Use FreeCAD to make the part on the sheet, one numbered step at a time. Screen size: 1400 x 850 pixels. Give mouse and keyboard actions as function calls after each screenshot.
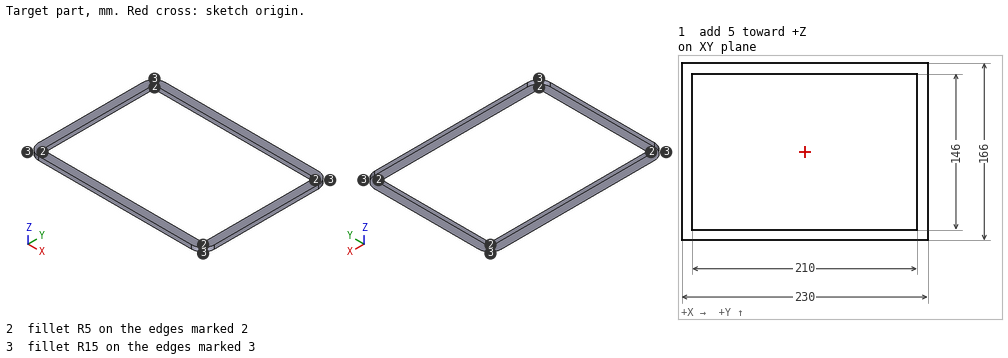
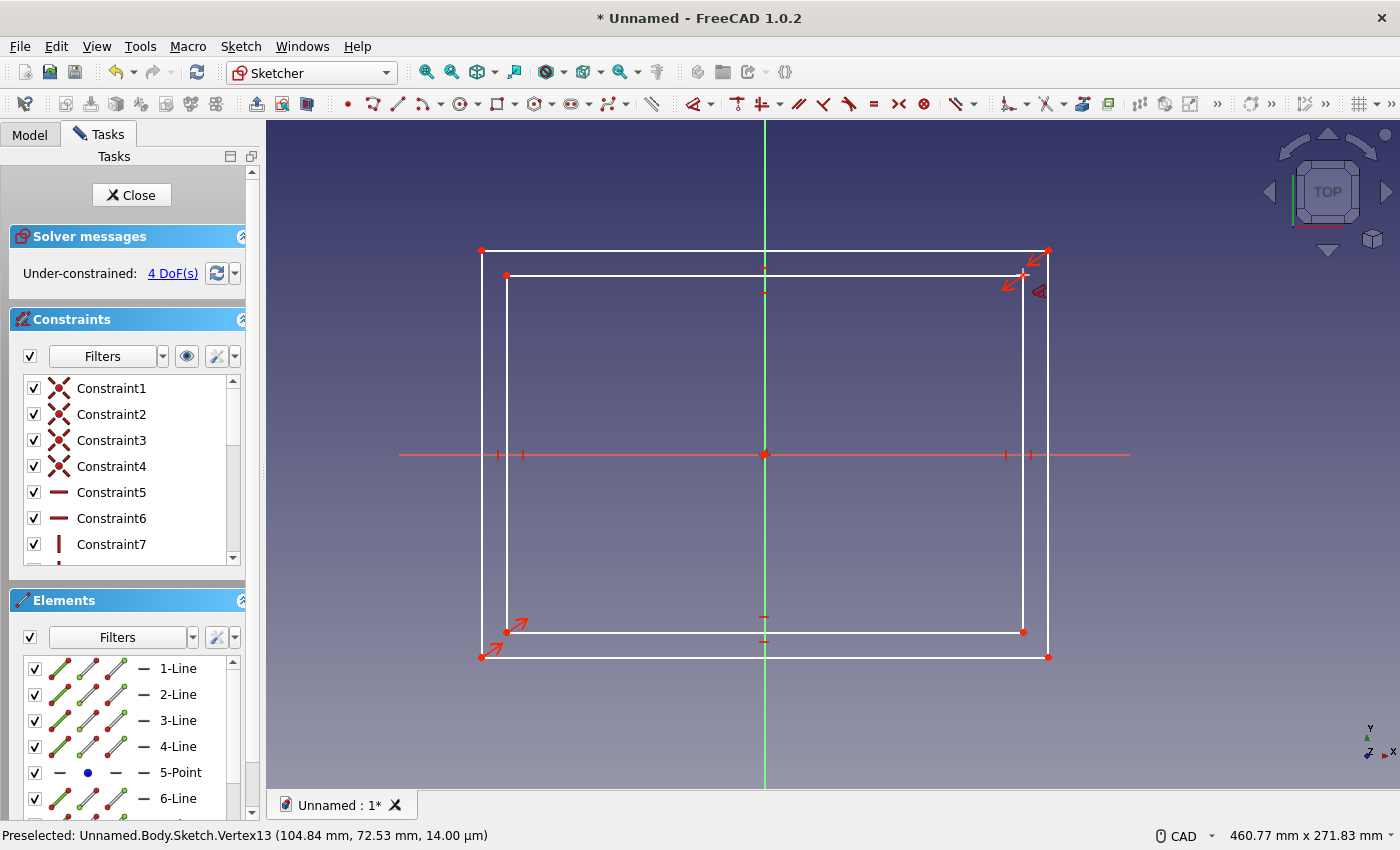
click(652, 658)
click(635, 692)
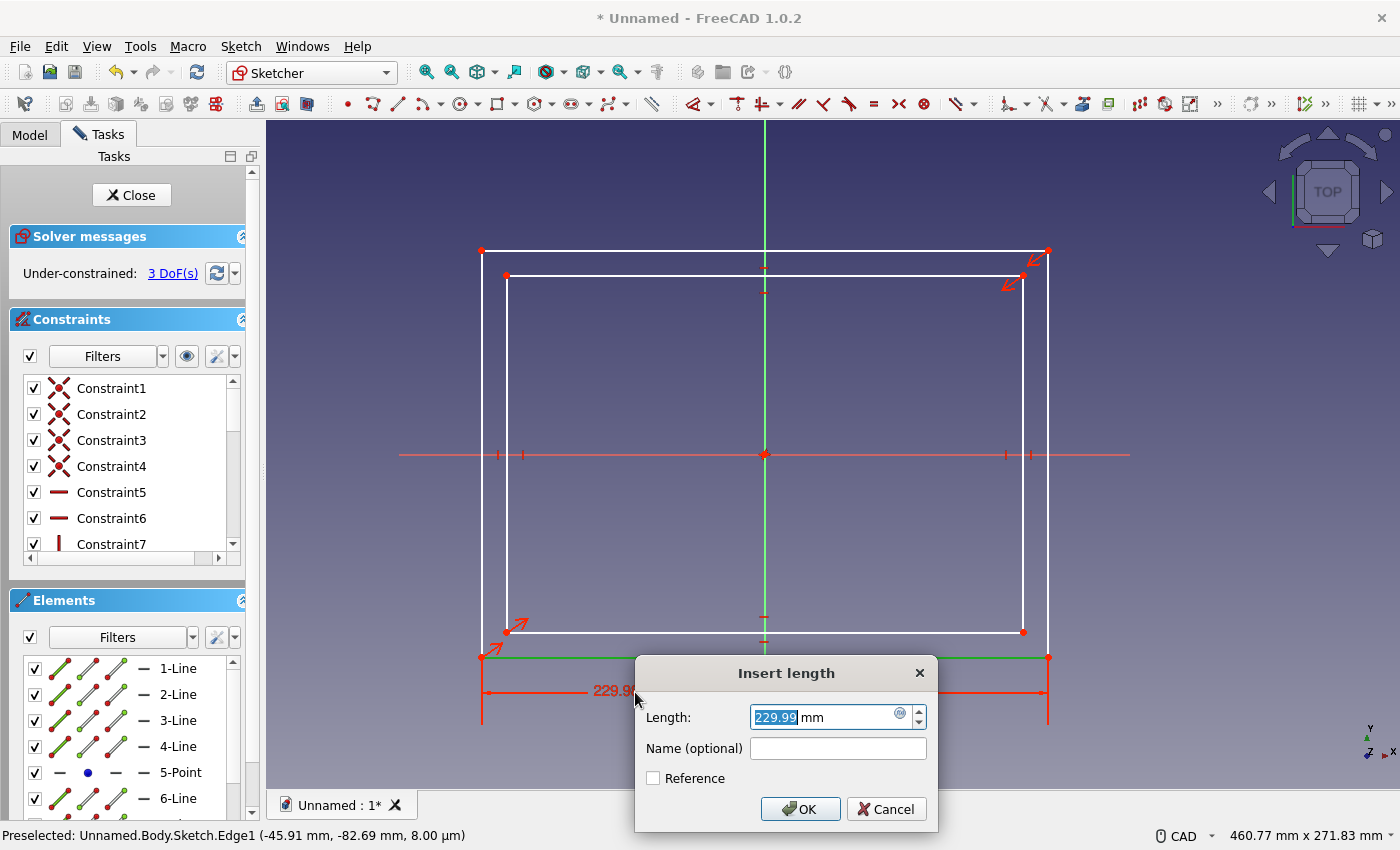
text(230)
key(Return)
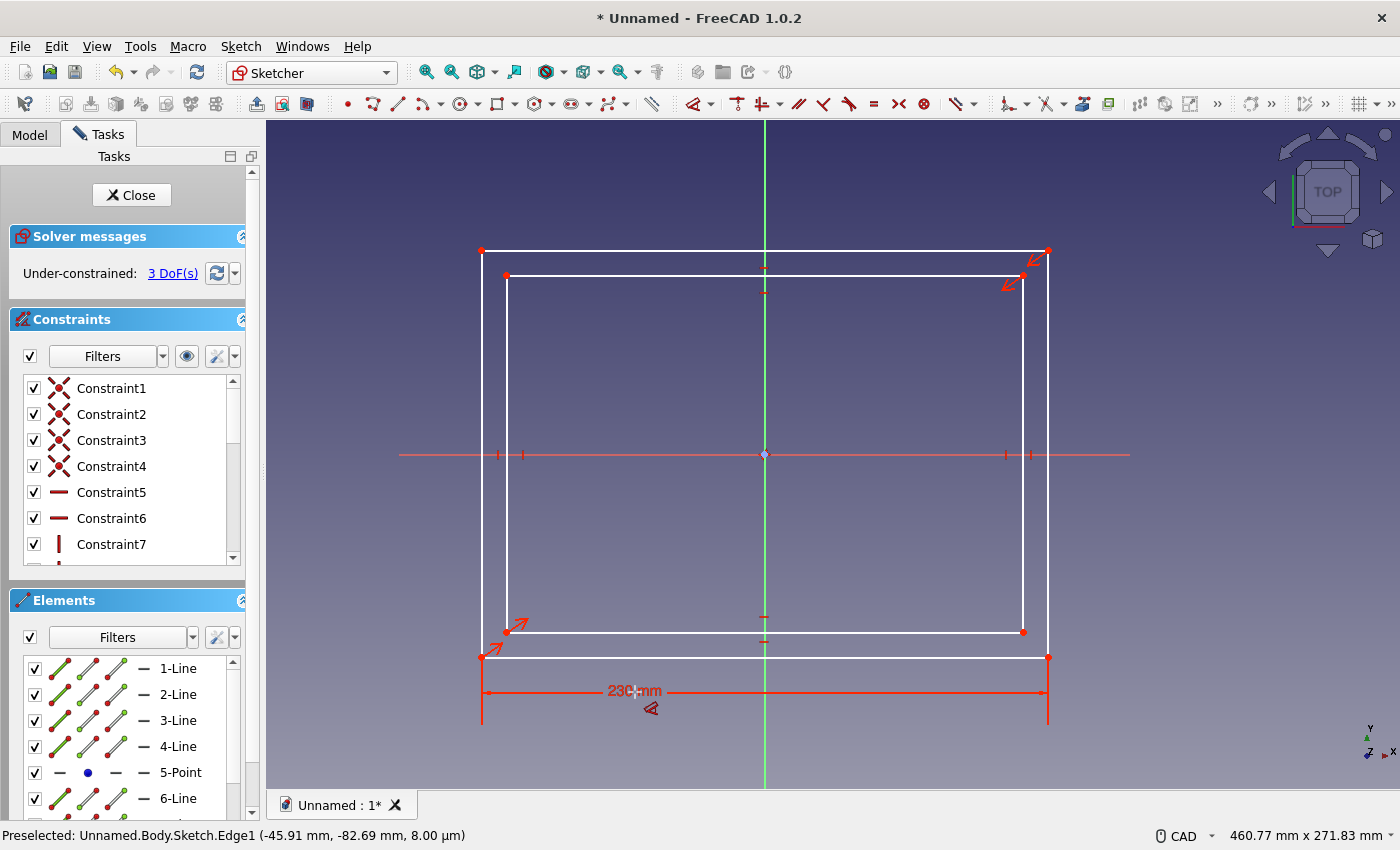
click(1048, 536)
click(1082, 361)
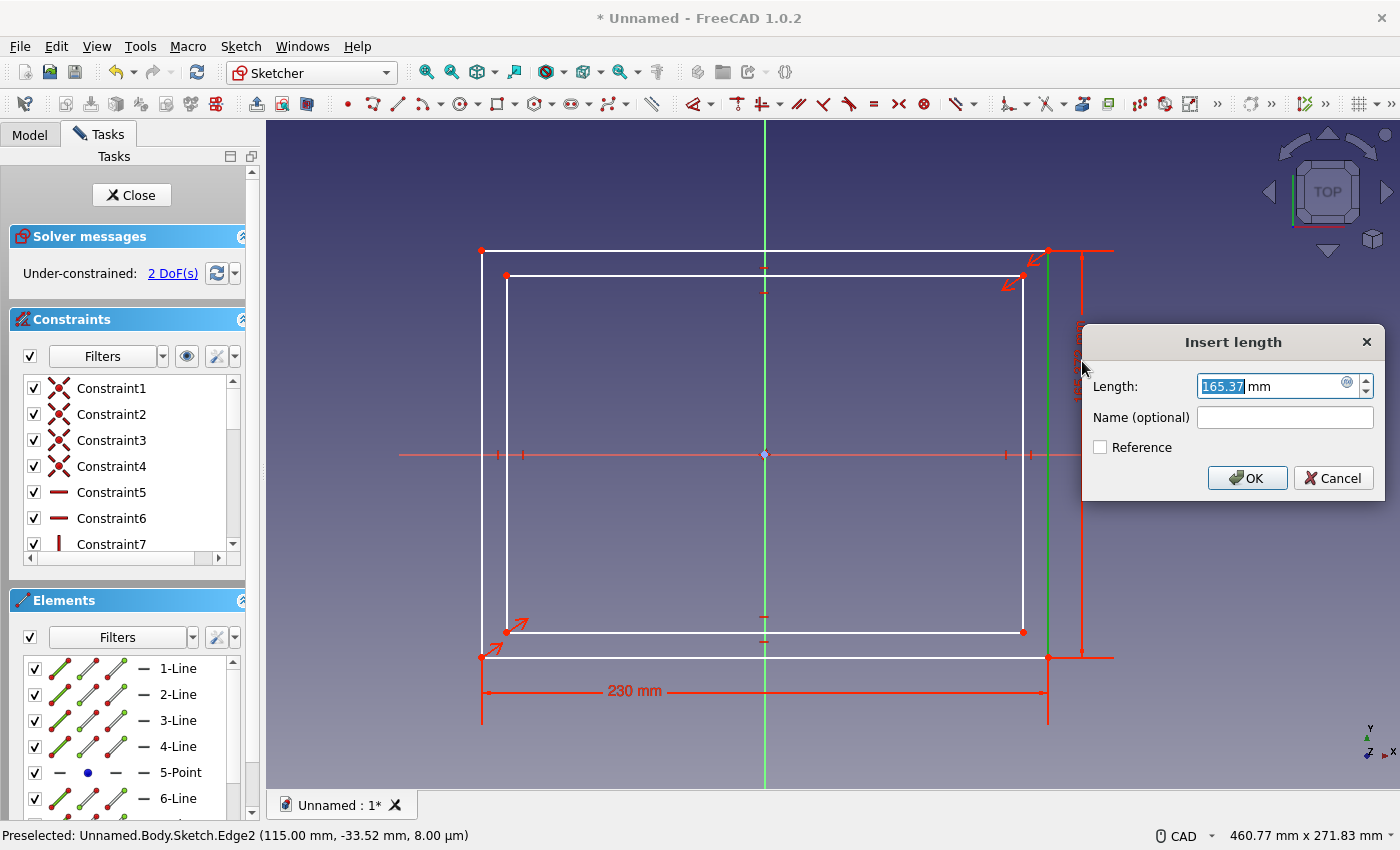
text(166)
key(Return)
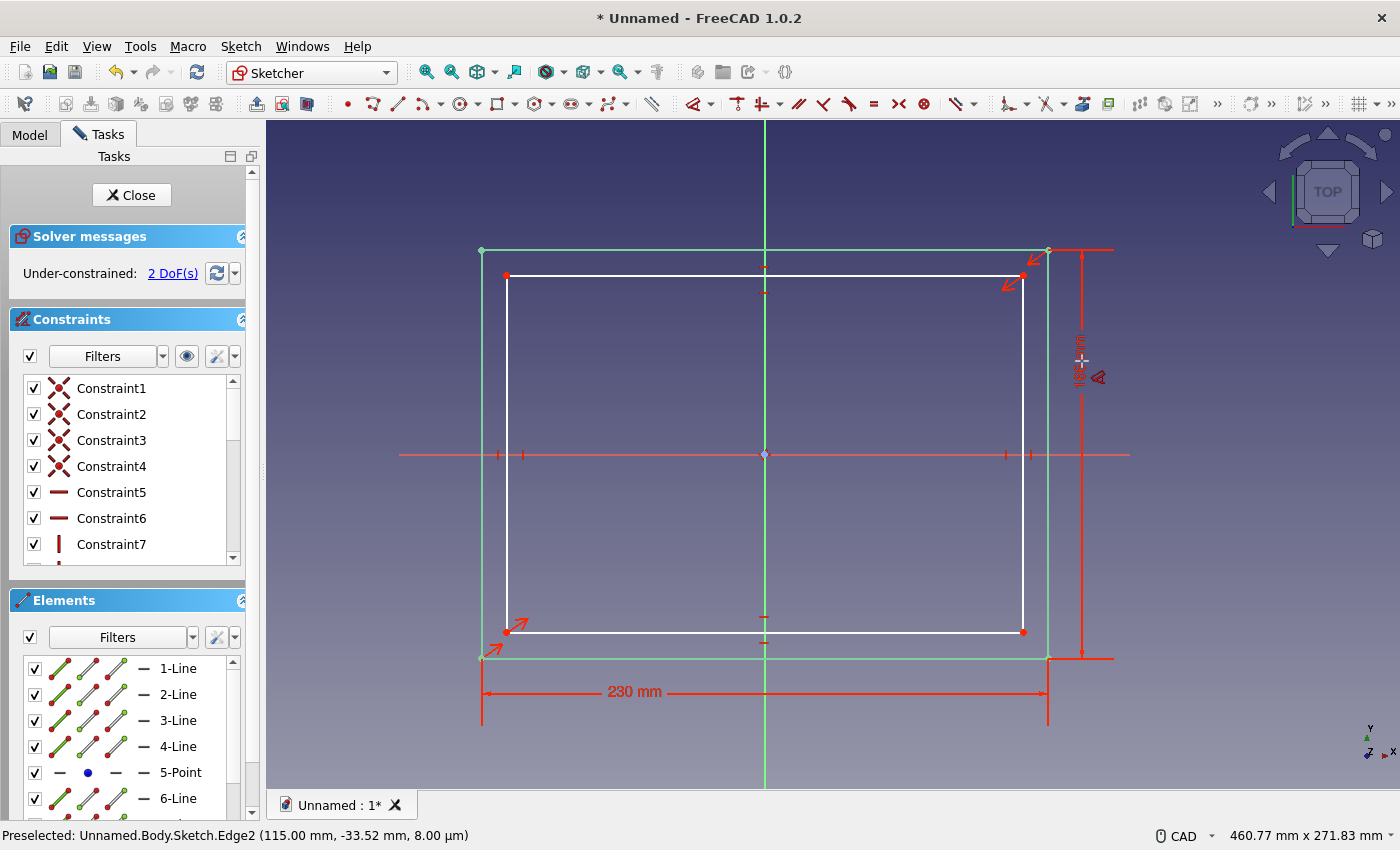
click(662, 633)
click(646, 599)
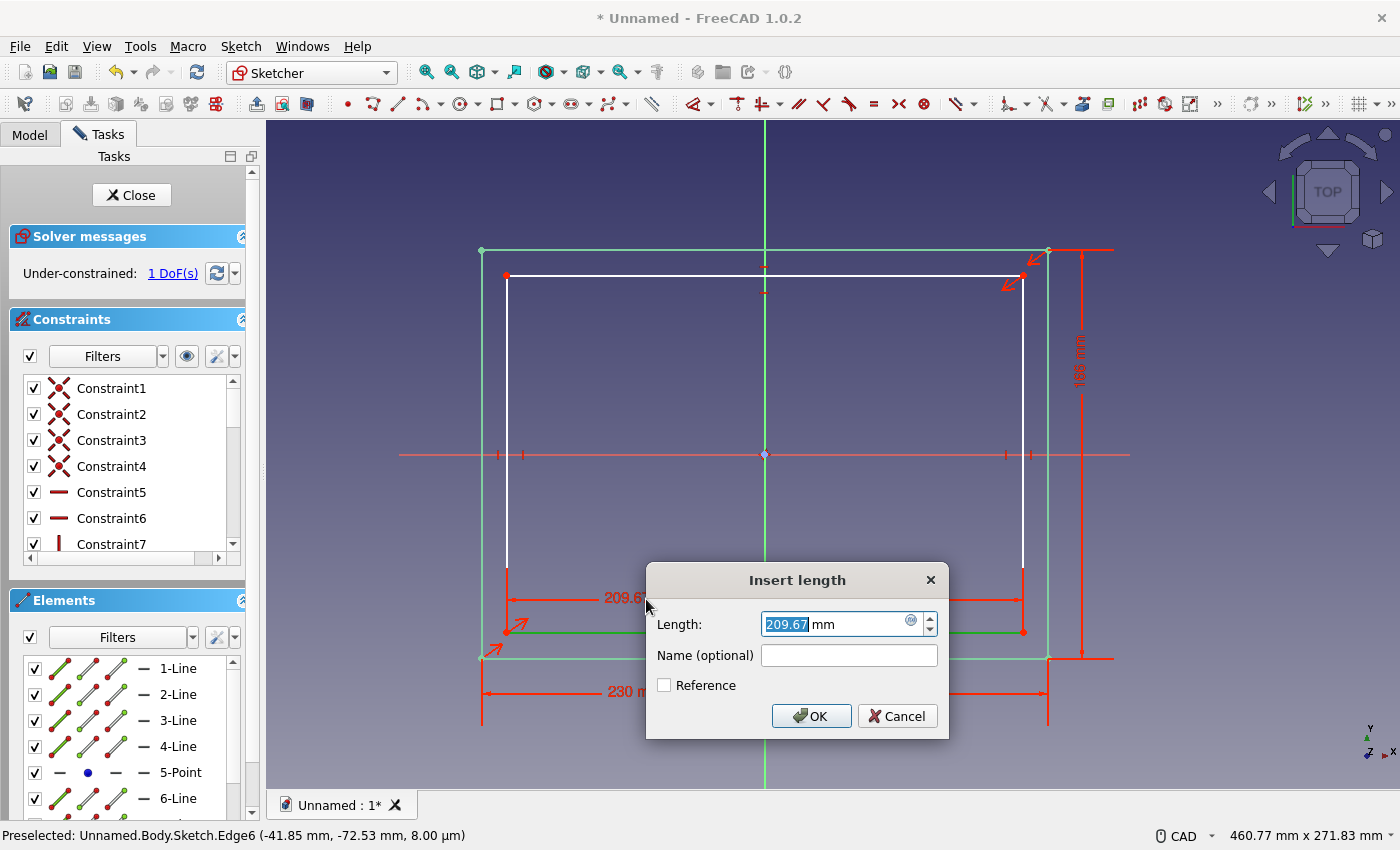
text(210)
key(Return)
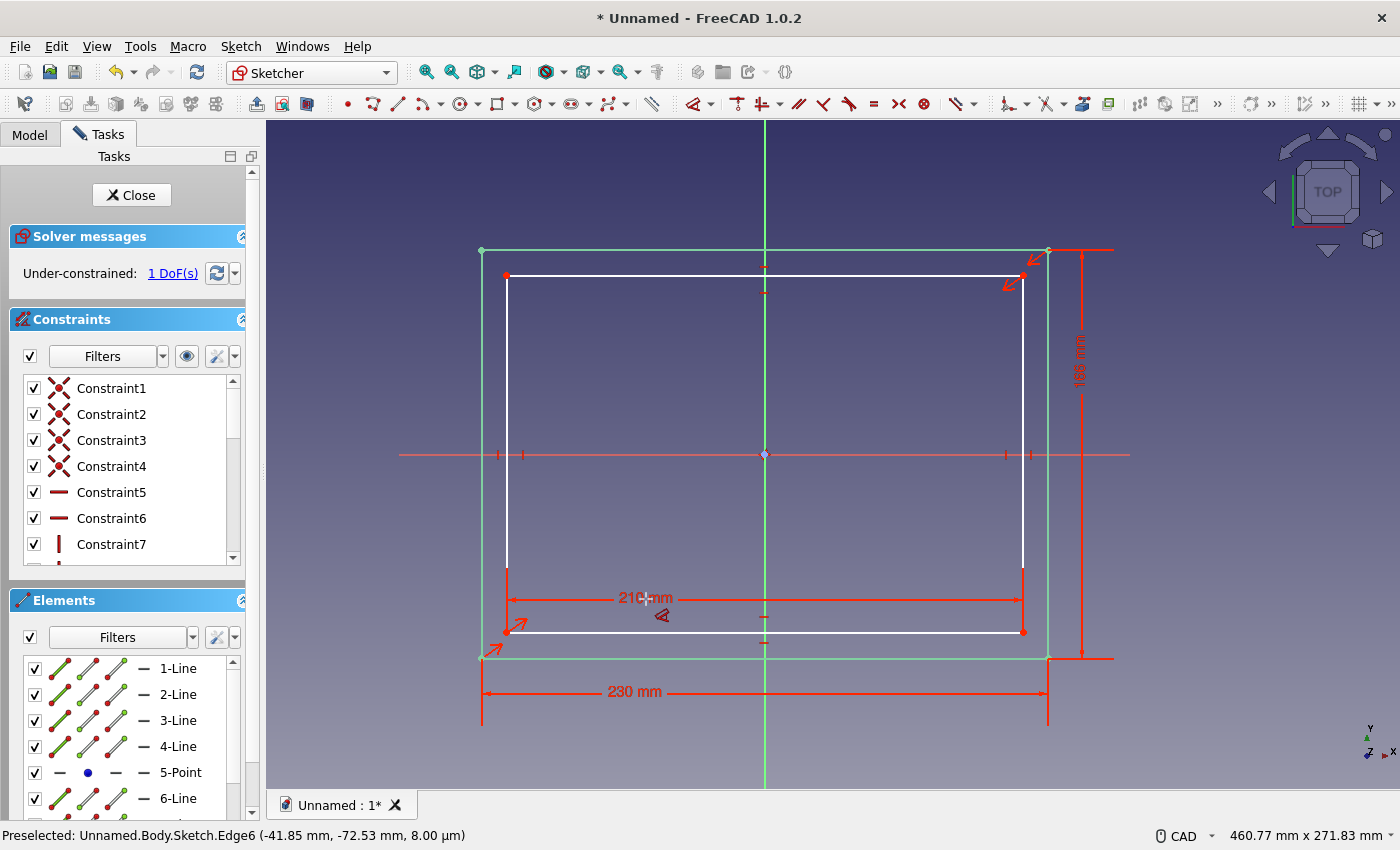
click(1023, 526)
click(989, 372)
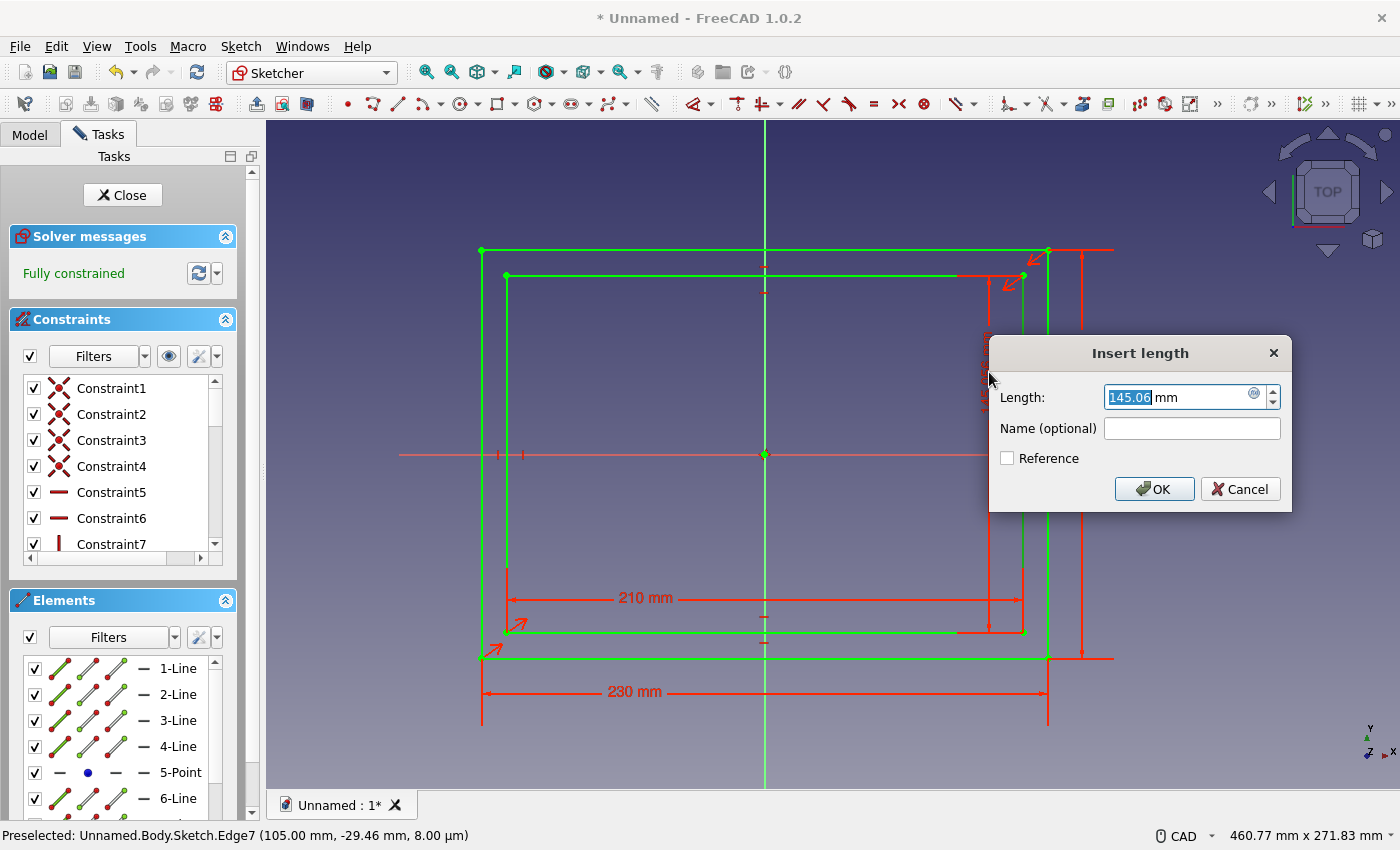
text(146)
key(Return)
key(Escape)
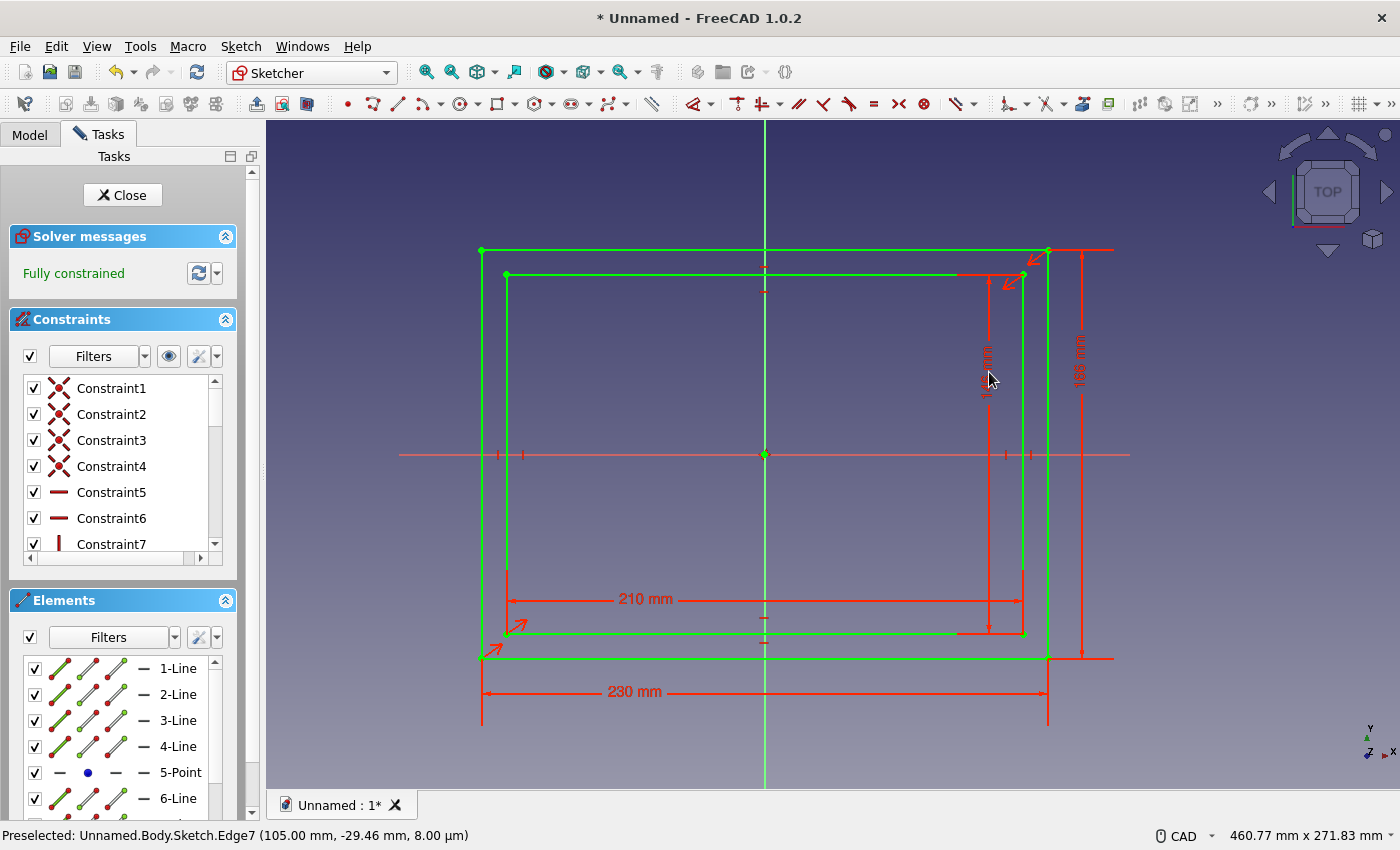
click(123, 195)